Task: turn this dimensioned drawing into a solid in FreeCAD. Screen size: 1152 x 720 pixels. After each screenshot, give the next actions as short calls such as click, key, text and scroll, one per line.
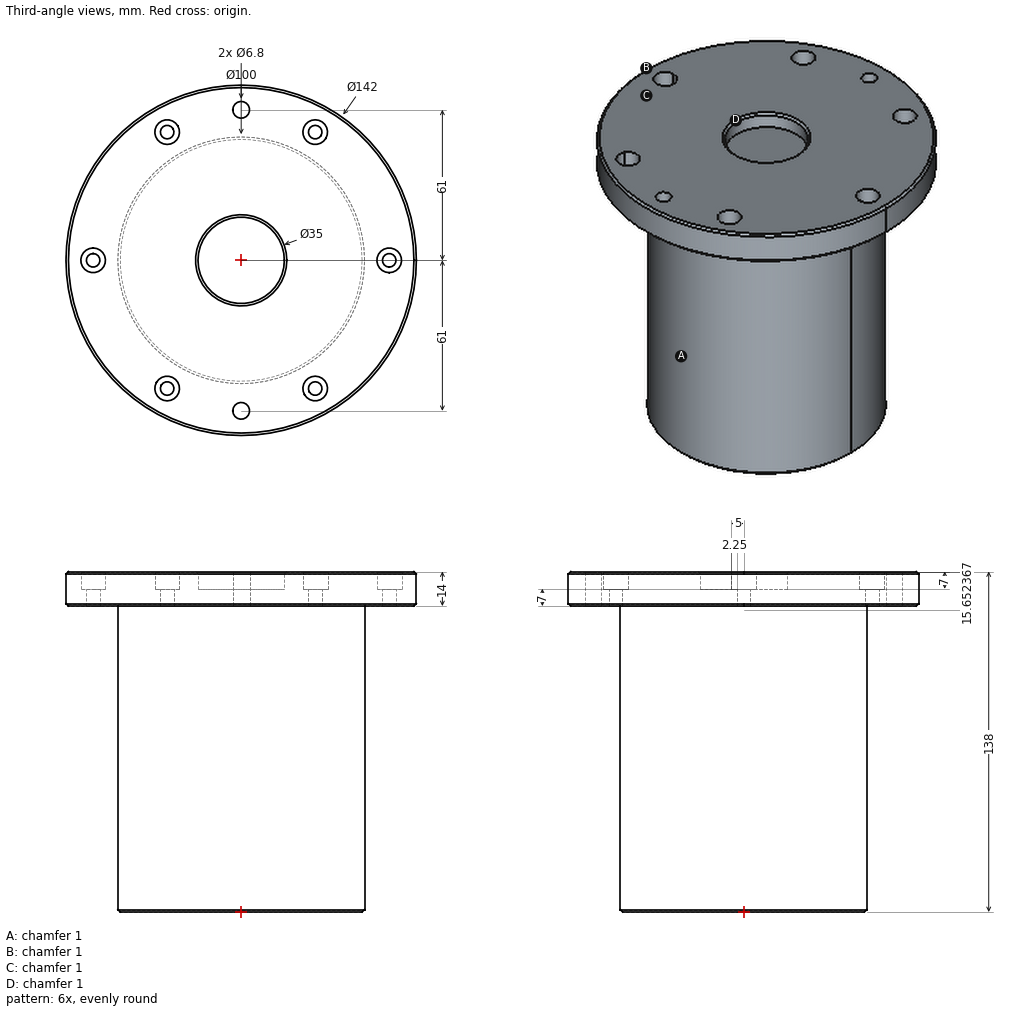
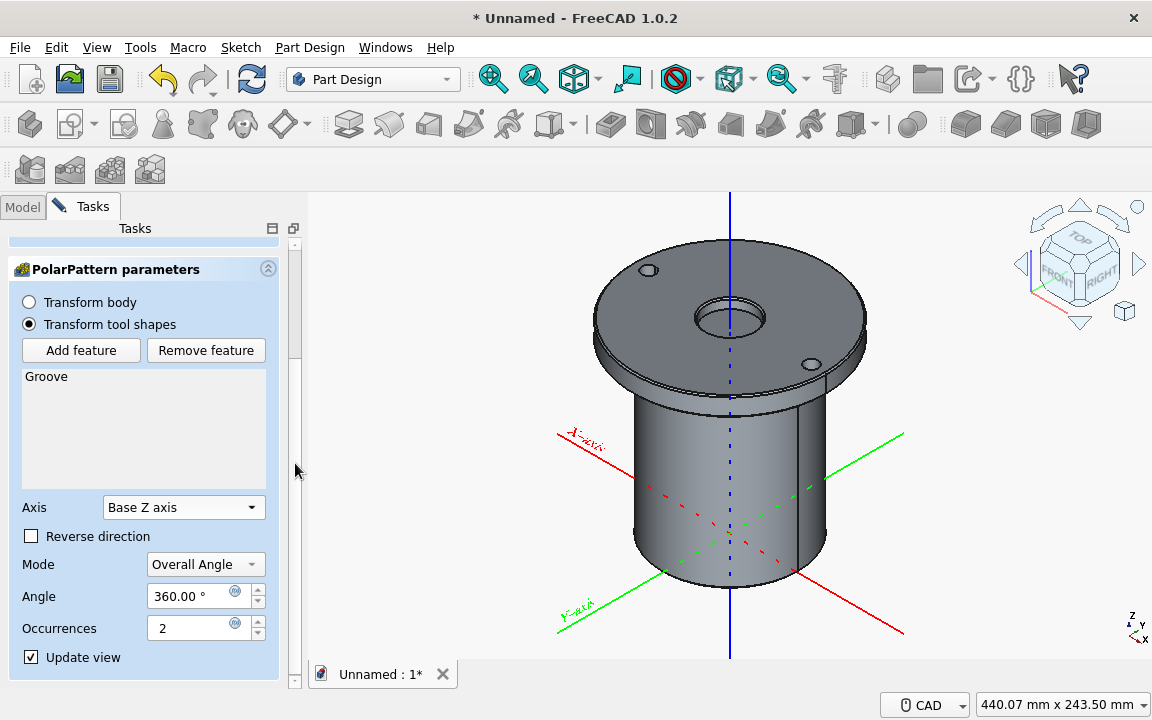
triple_click(198, 628)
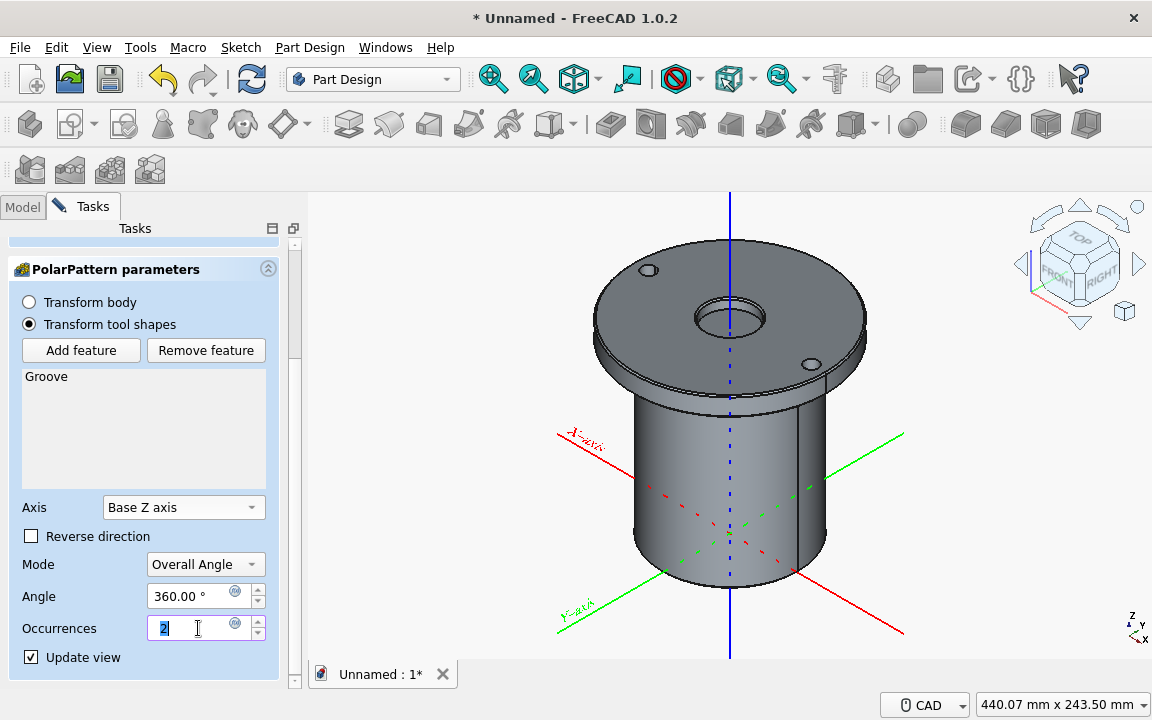
text(6)
key(Tab)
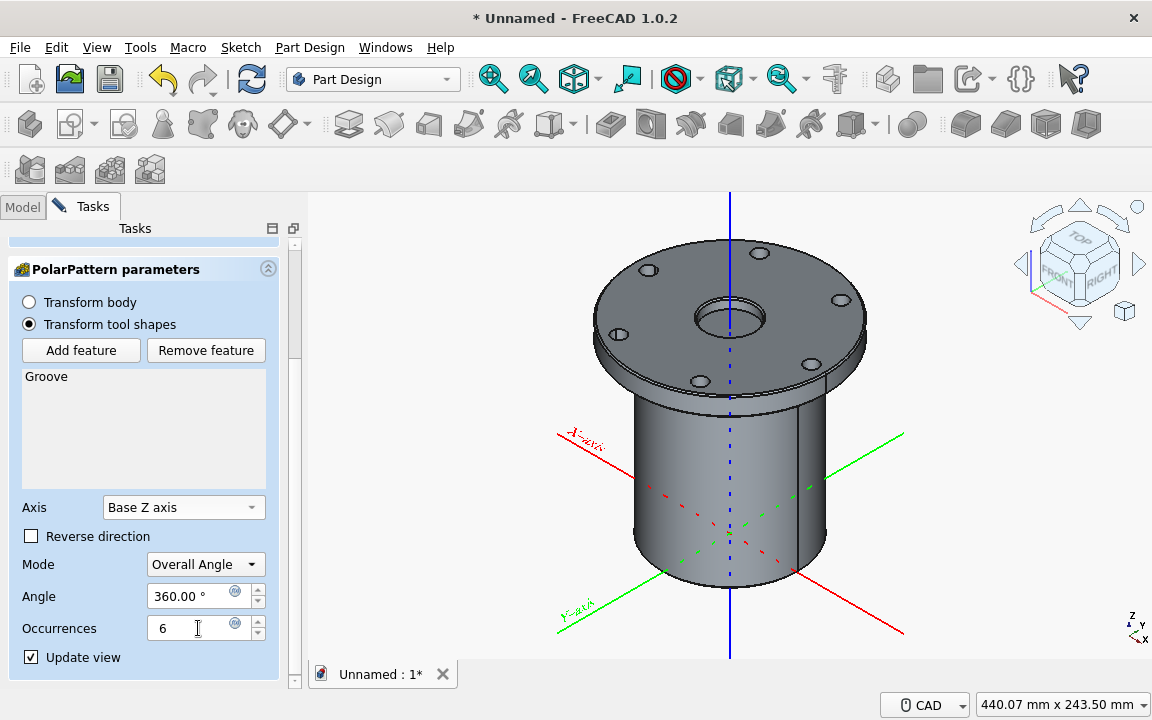
scroll(295, 463, up, 4)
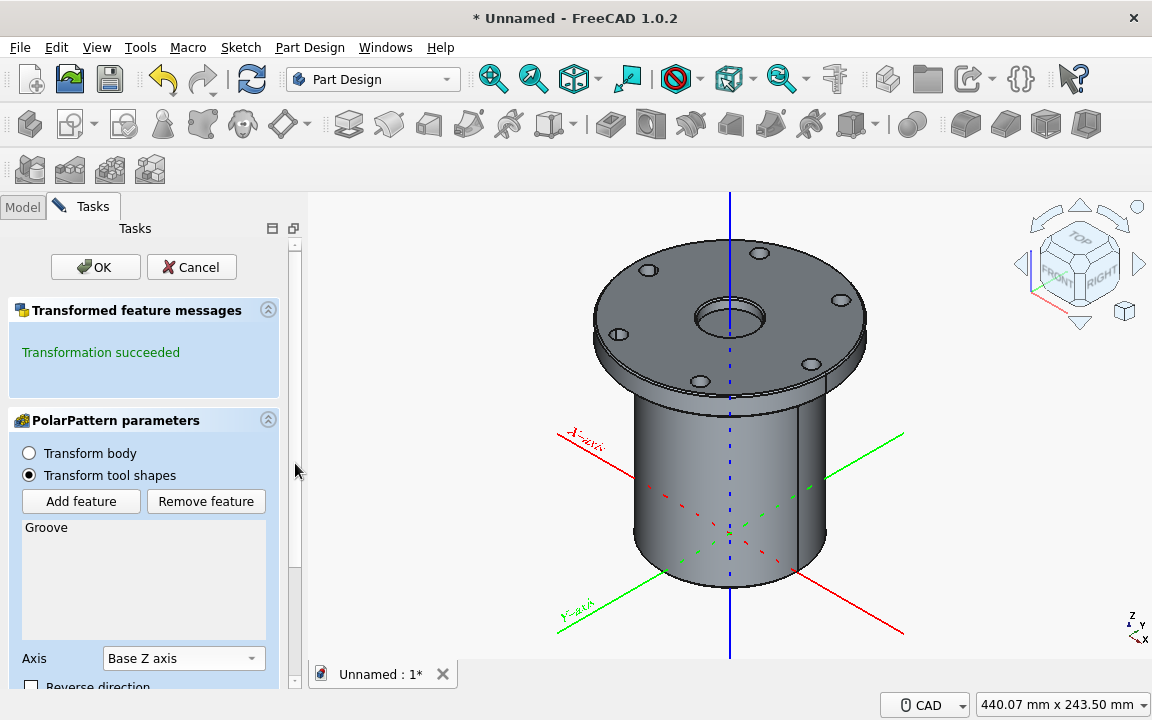
click(96, 267)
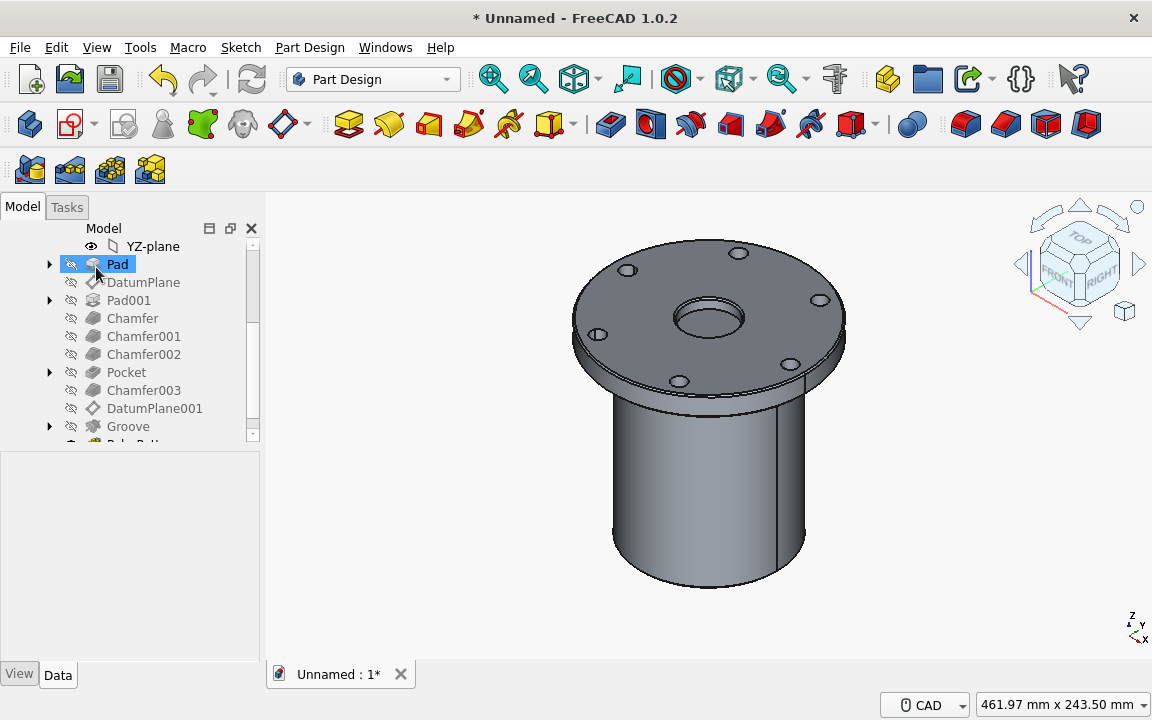
click(790, 332)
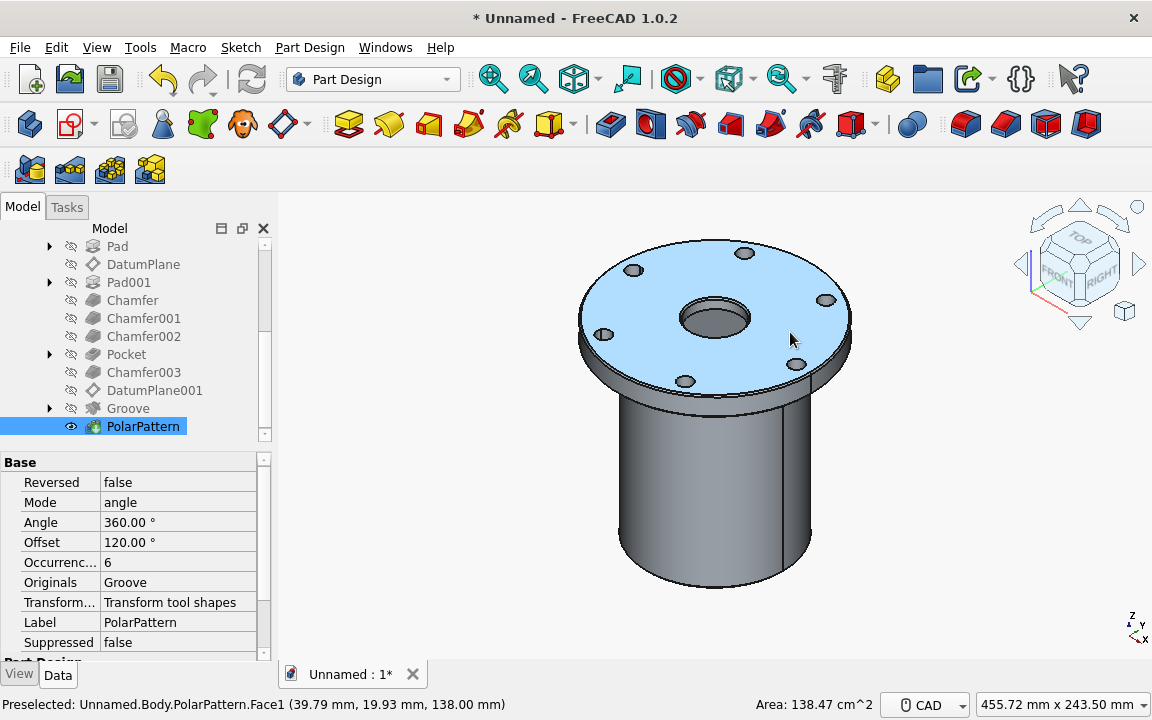
click(70, 124)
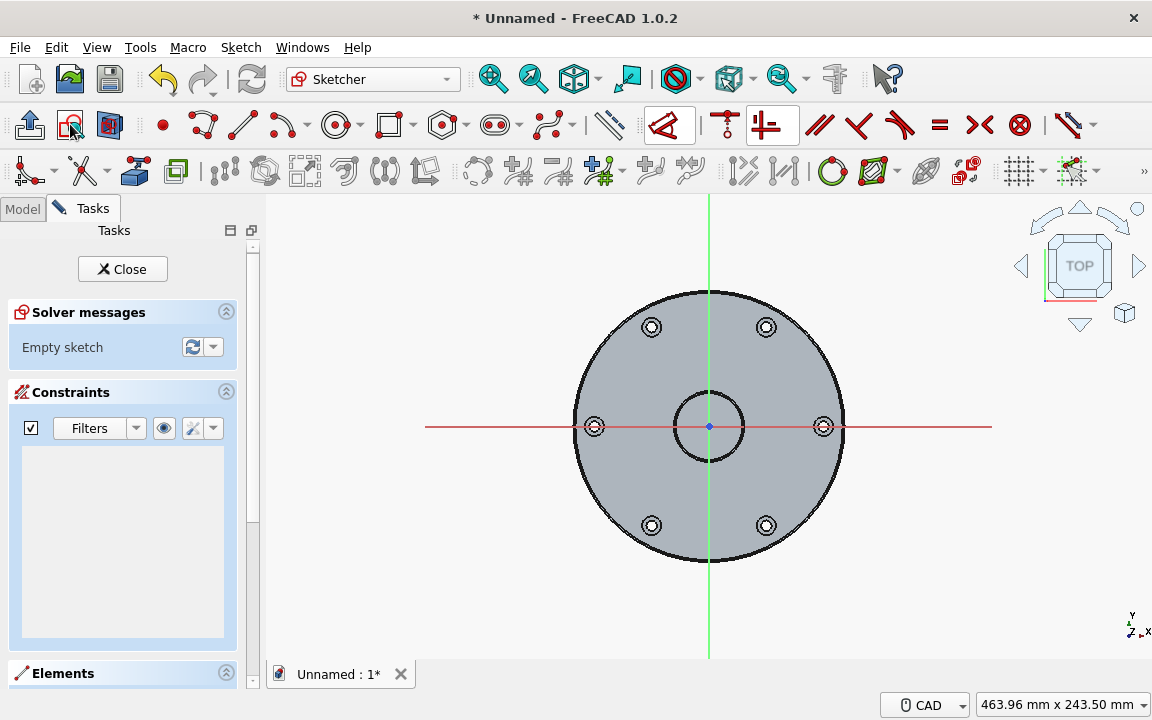
key(g)
key(c)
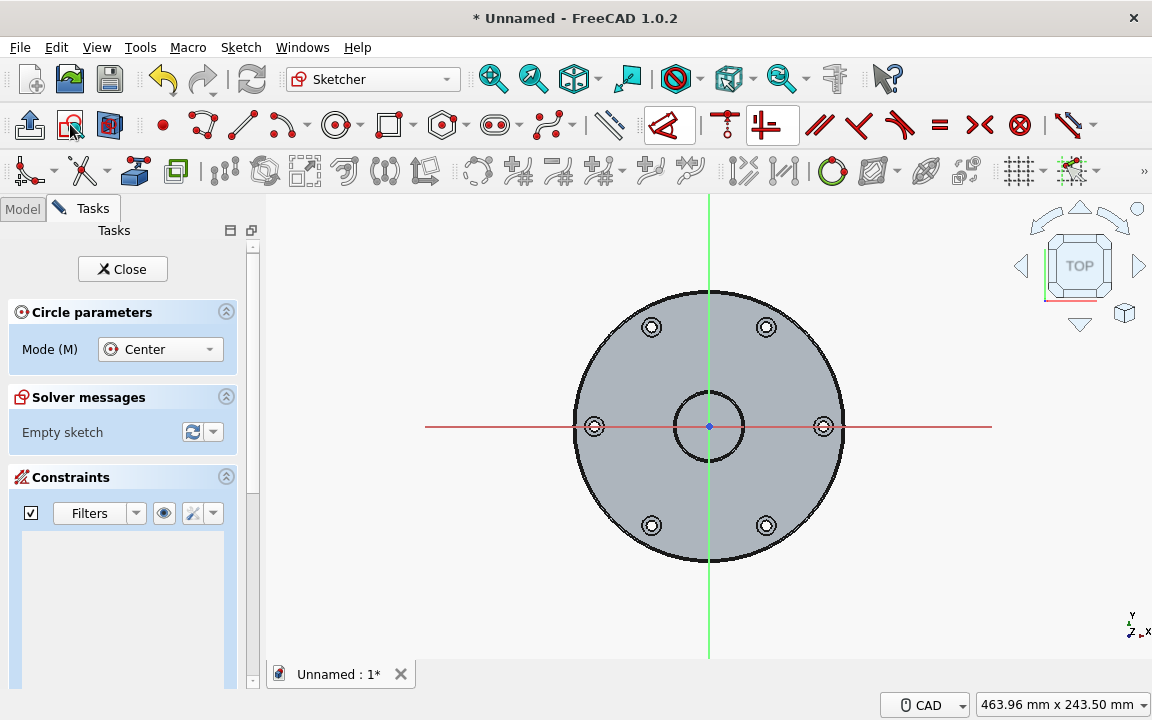
scroll(709, 310, up, 7)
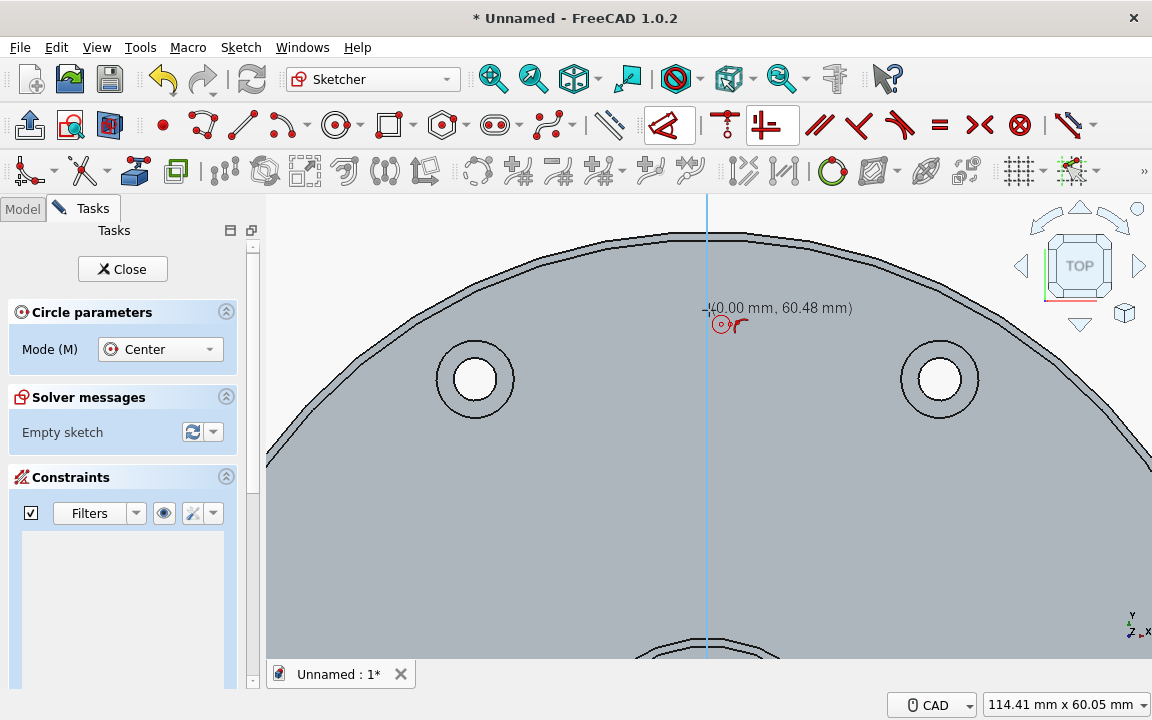
scroll(612, 273, down, 6)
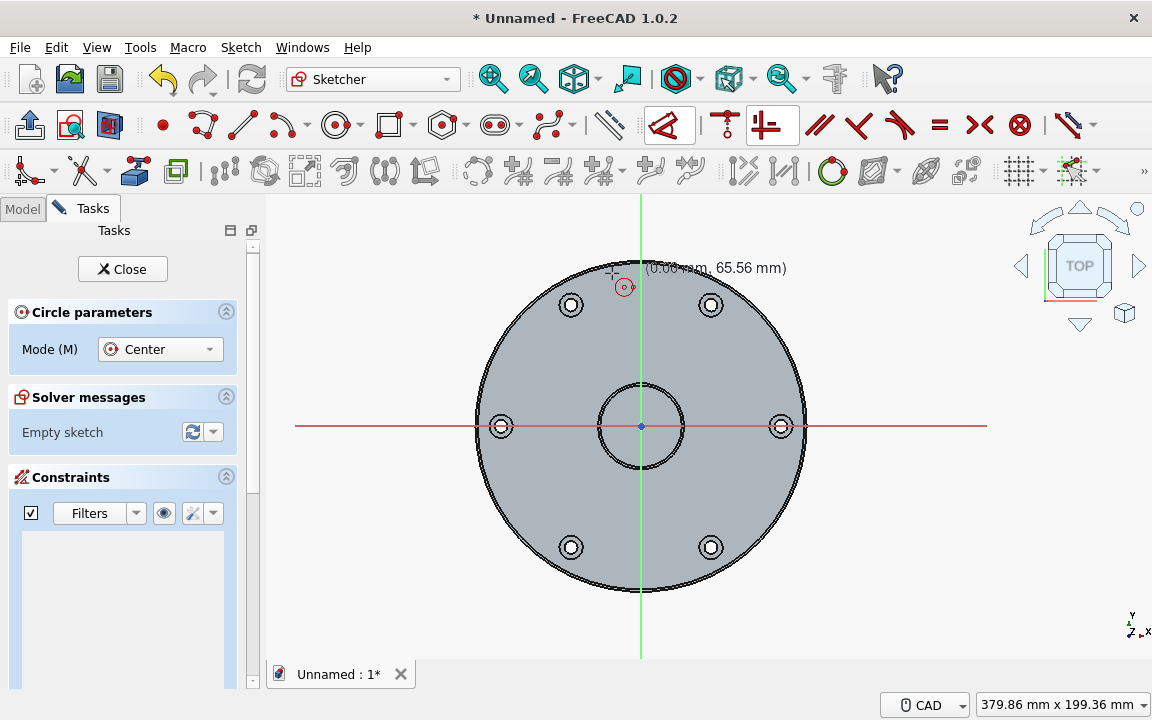
click(641, 284)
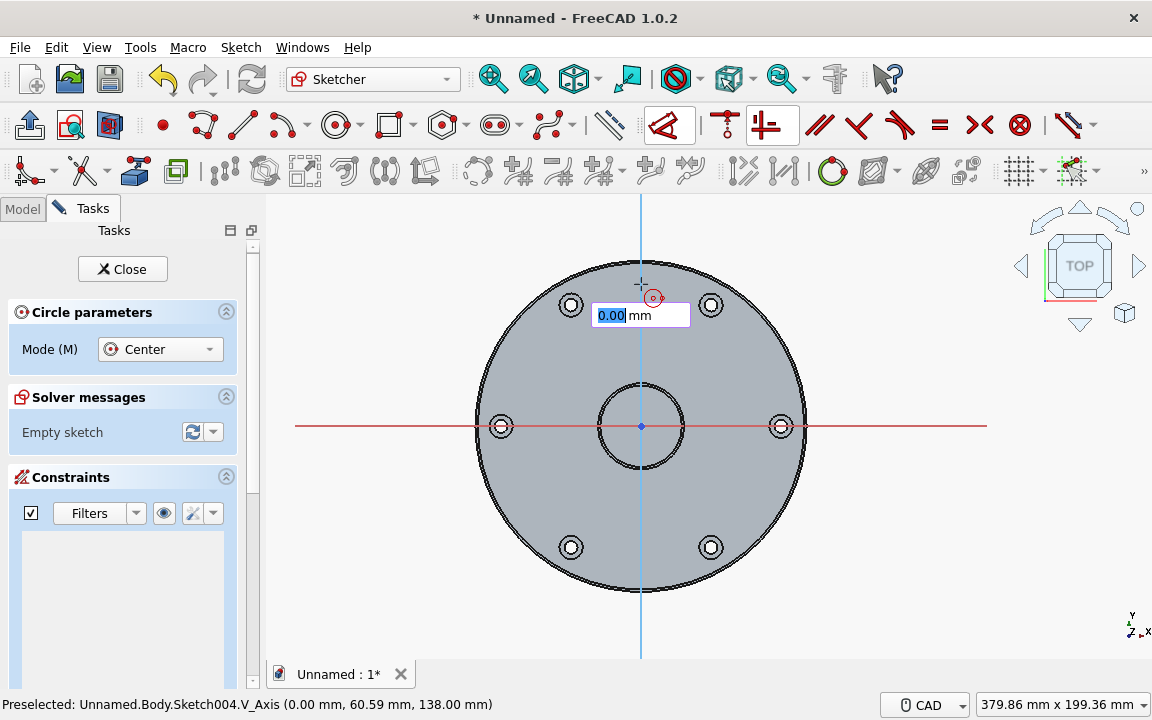
scroll(648, 281, up, 4)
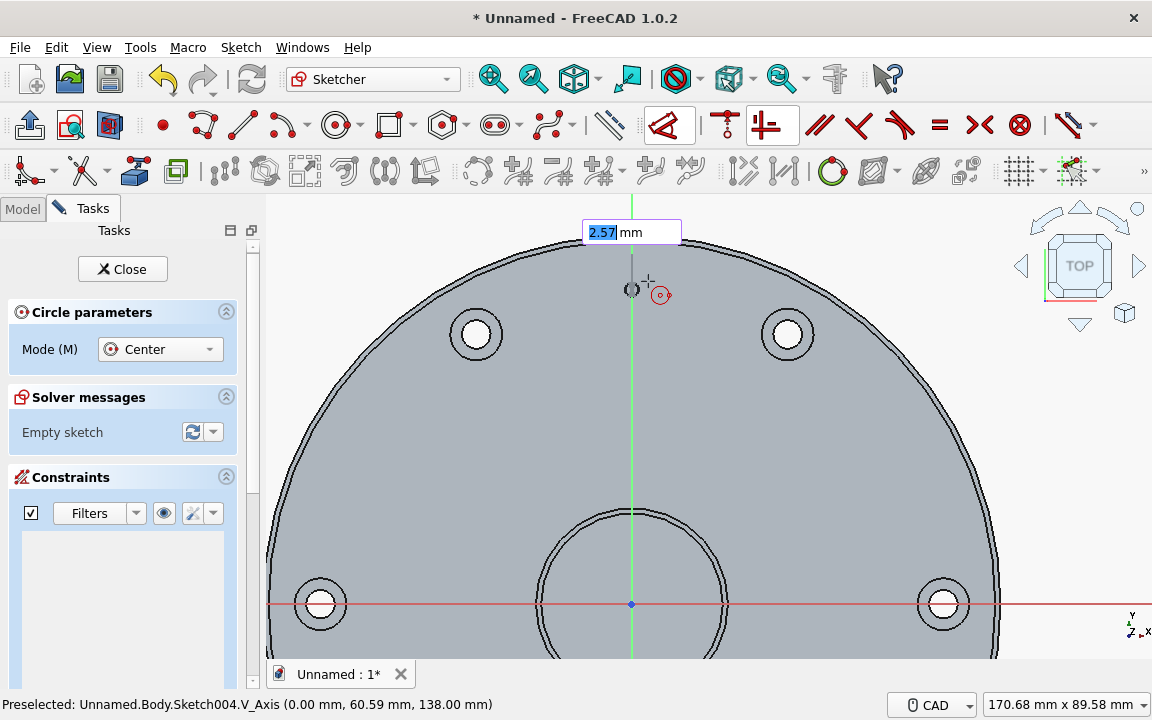
click(649, 282)